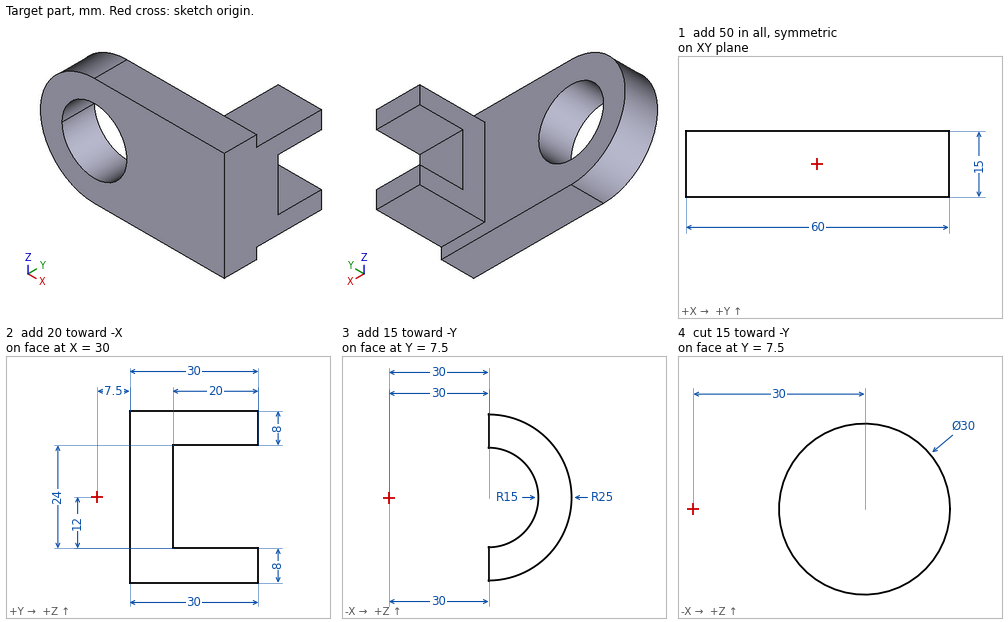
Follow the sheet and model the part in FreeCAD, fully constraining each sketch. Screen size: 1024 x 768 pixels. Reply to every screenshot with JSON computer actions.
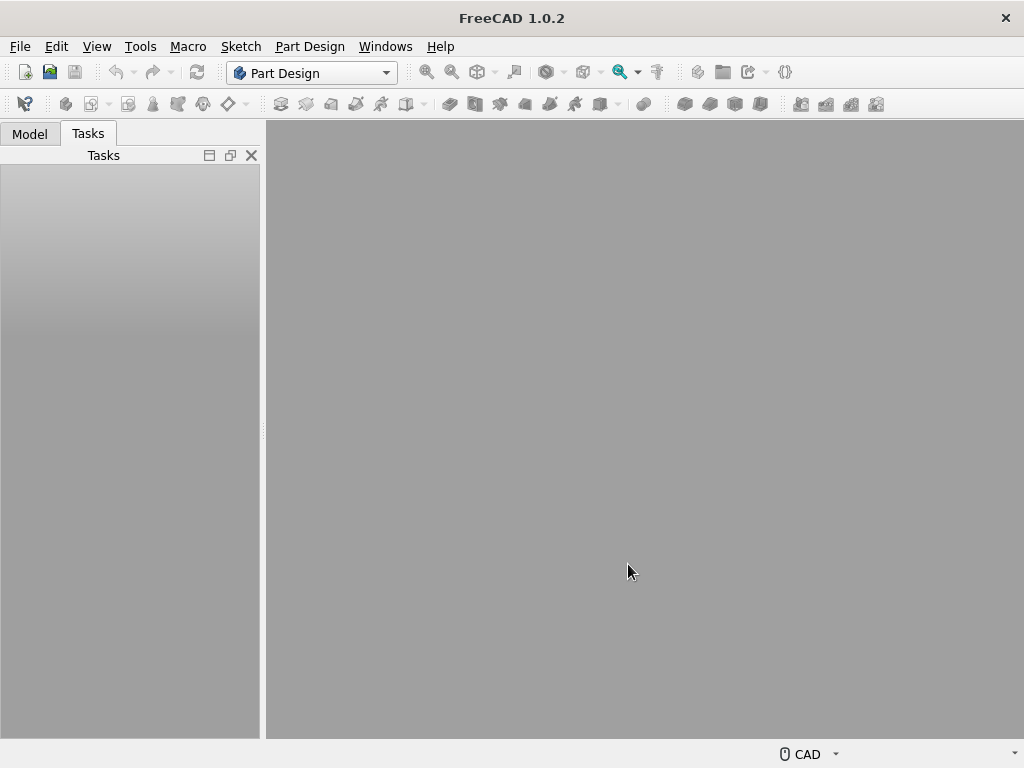
{"action": "left_click", "coordinate": [25, 72]}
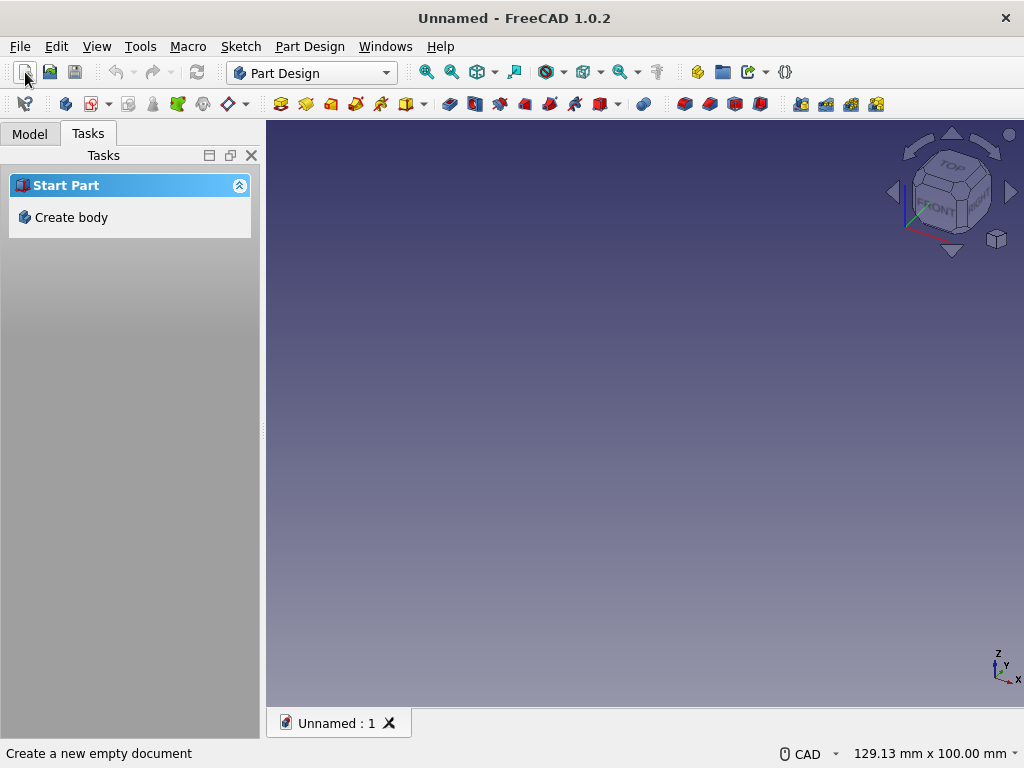
{"action": "left_click", "coordinate": [90, 104]}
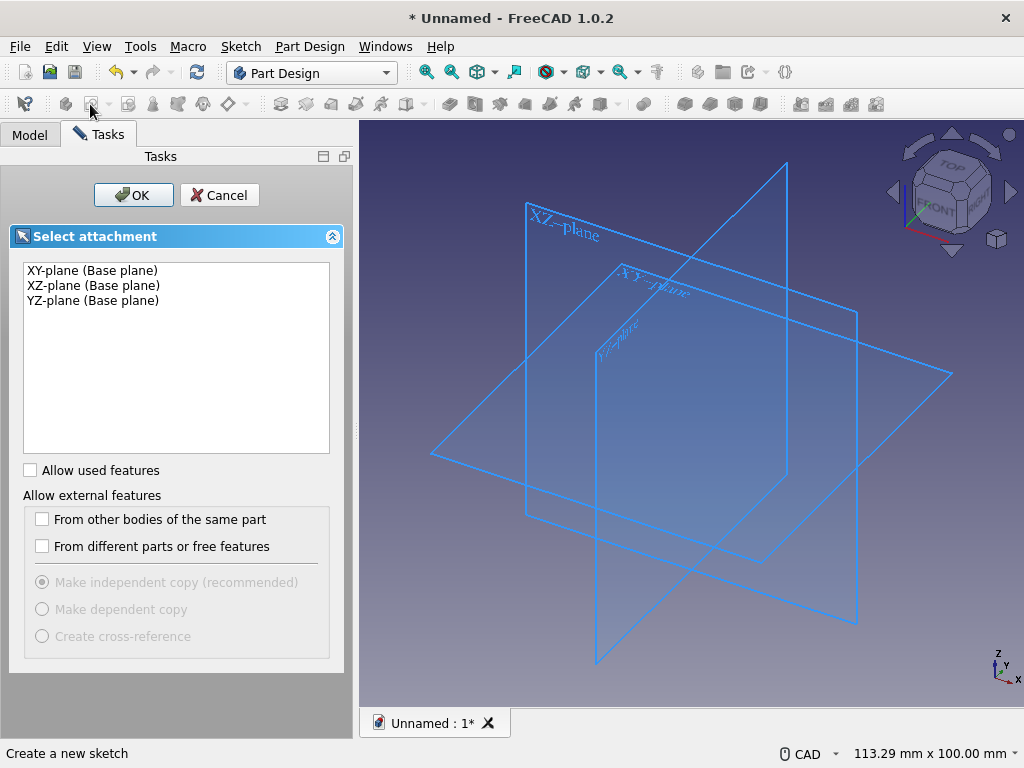
{"action": "left_click", "coordinate": [84, 270]}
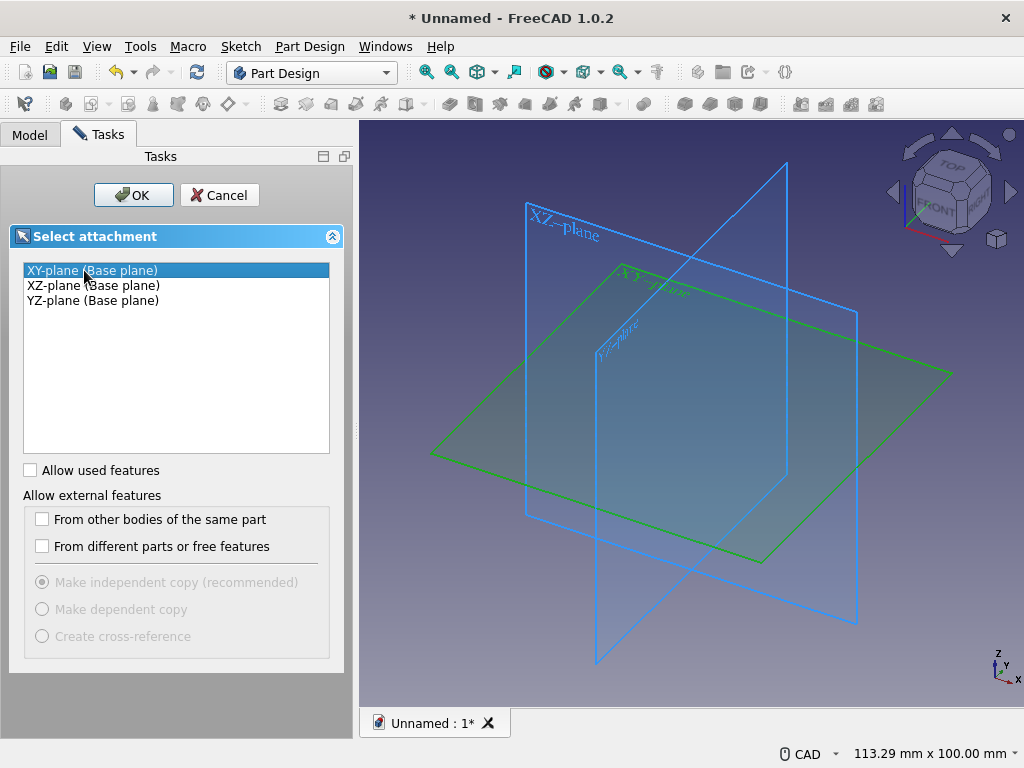
{"action": "left_click", "coordinate": [134, 195]}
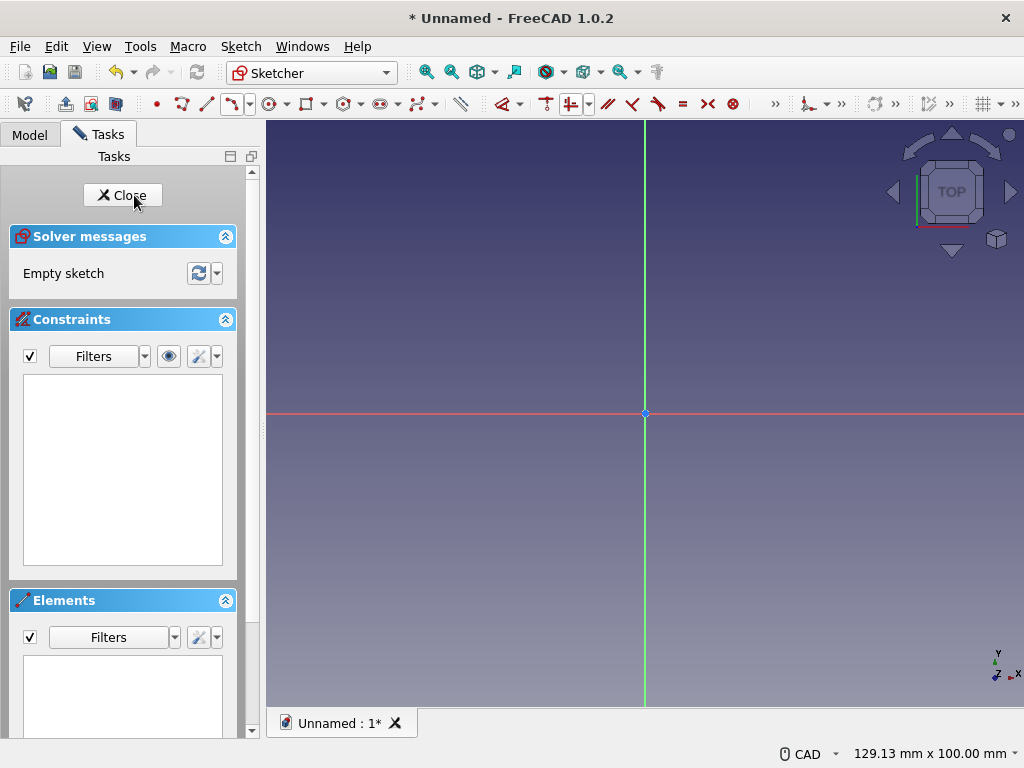
{"action": "key", "text": "g v"}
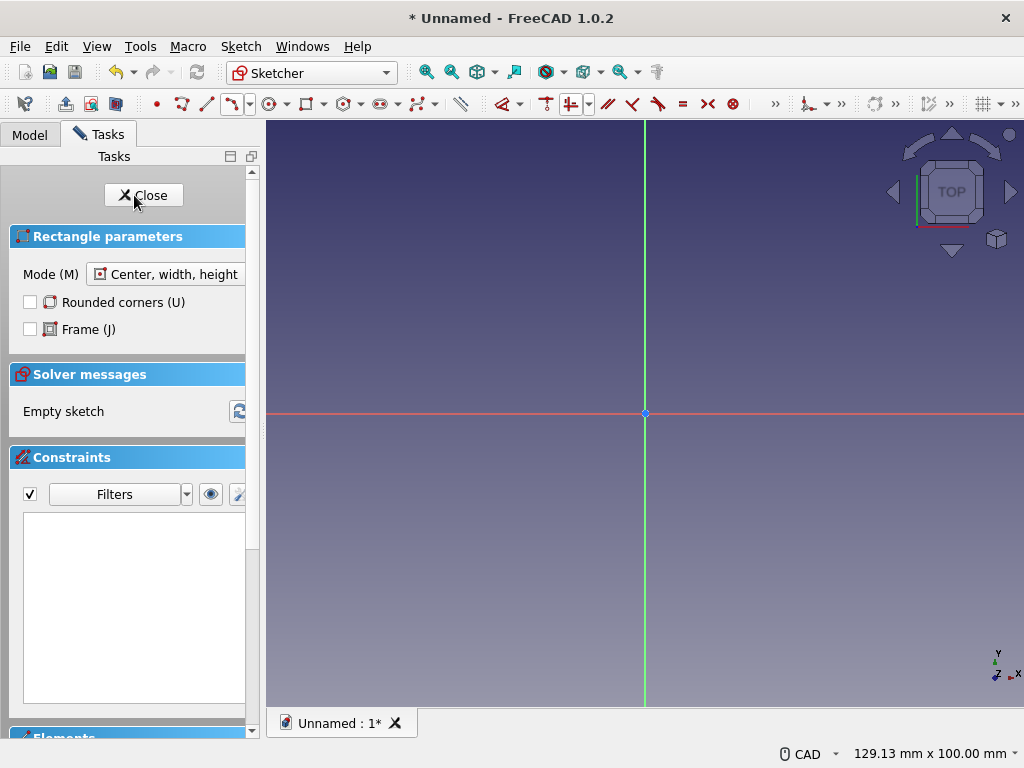
{"action": "left_click", "coordinate": [645, 414]}
{"action": "mouse_move", "coordinate": [821, 369]}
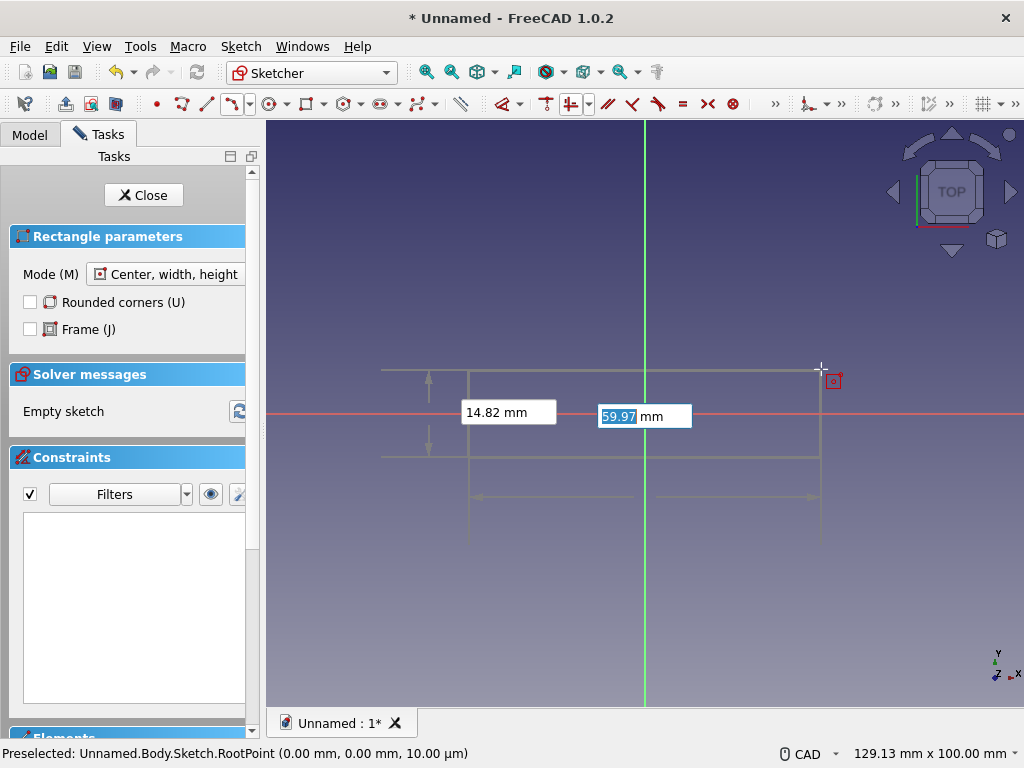
{"action": "type", "text": "60"}
{"action": "key", "text": "Tab"}
{"action": "type", "text": "15"}
{"action": "key", "text": "Return"}
{"action": "key", "text": "Escape"}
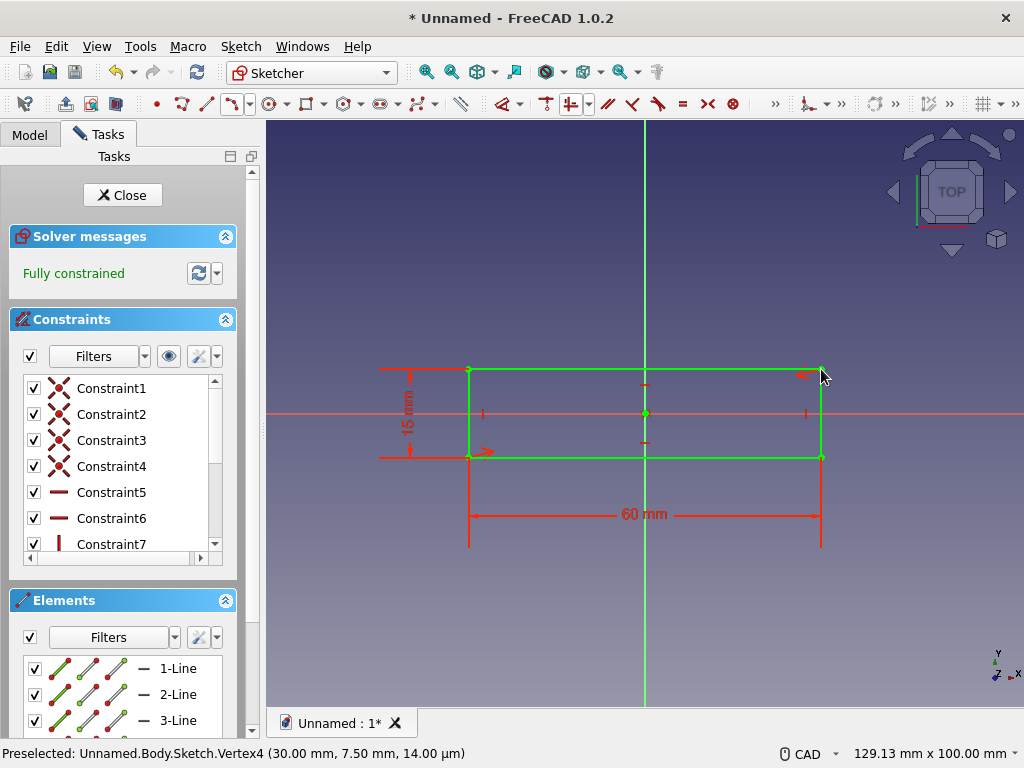
{"action": "left_click", "coordinate": [123, 195]}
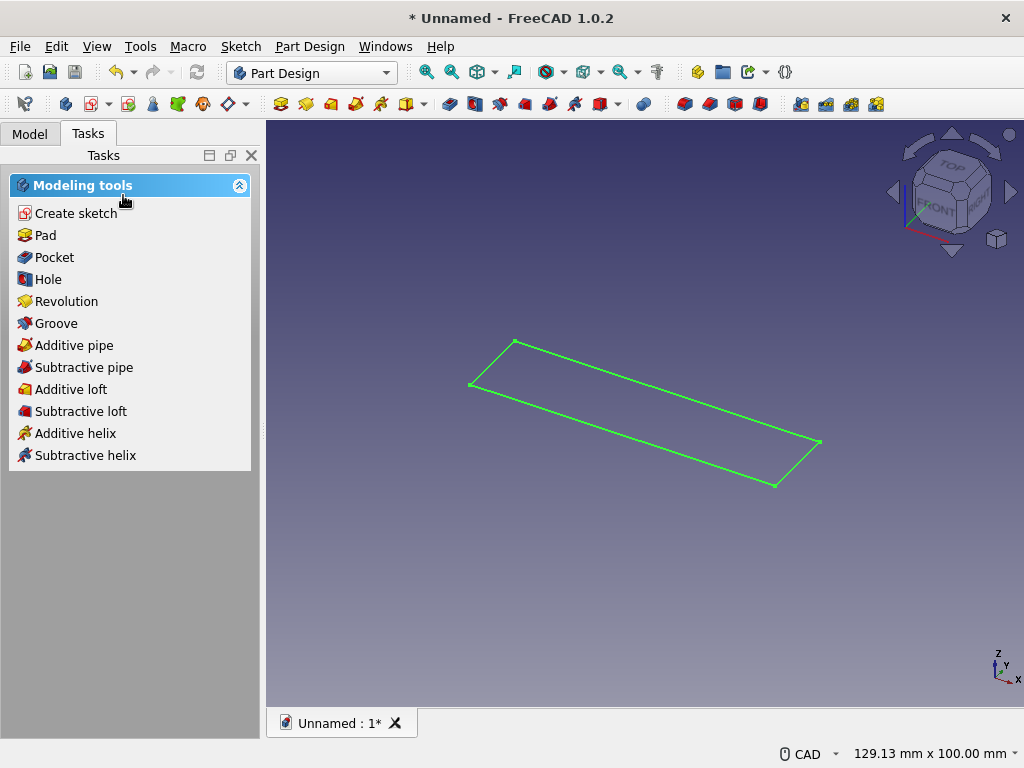
{"action": "left_click", "coordinate": [281, 104]}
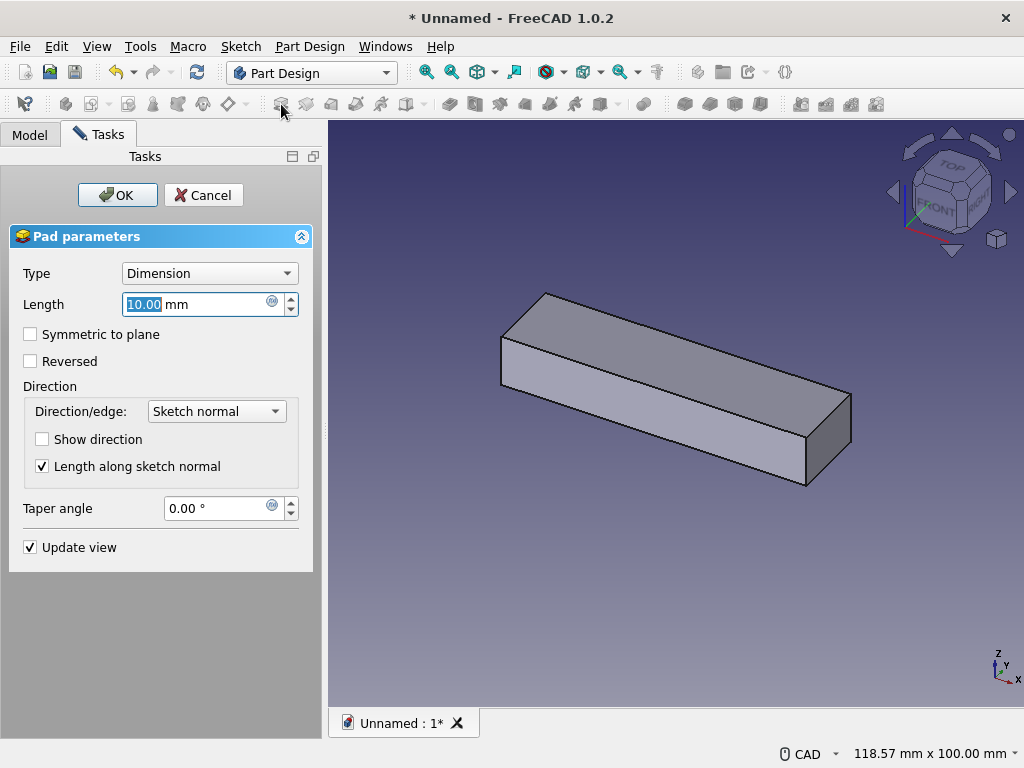
{"action": "type", "text": "50"}
{"action": "key", "text": "Tab"}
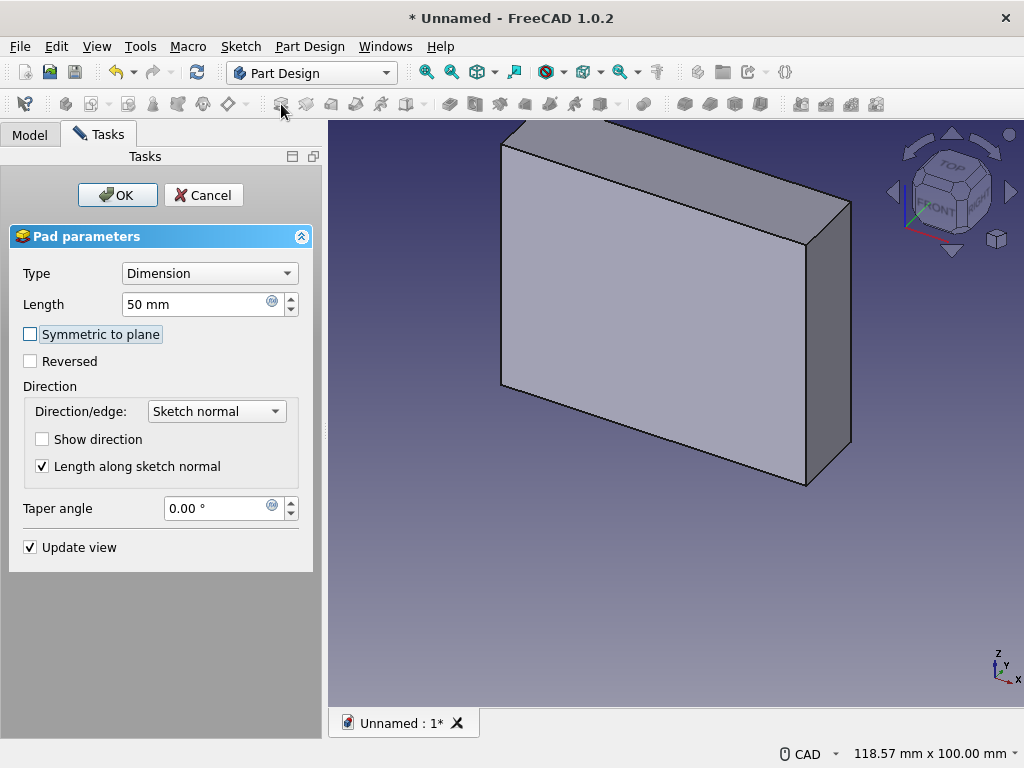
{"action": "left_click", "coordinate": [31, 334]}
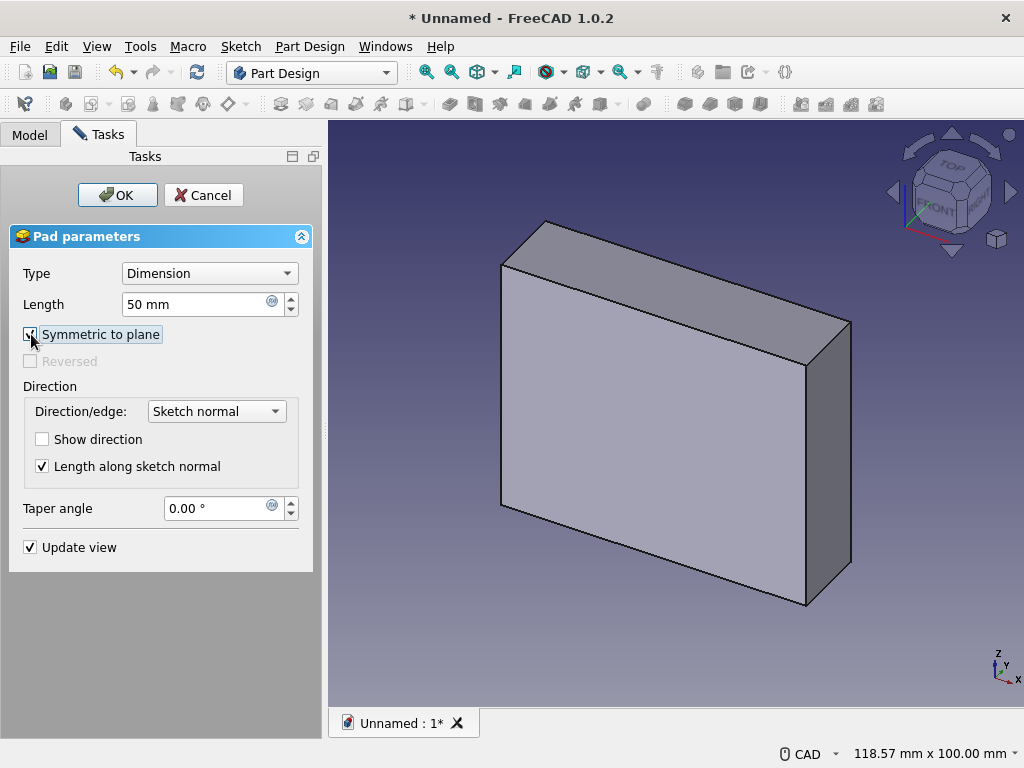
{"action": "left_click", "coordinate": [118, 195]}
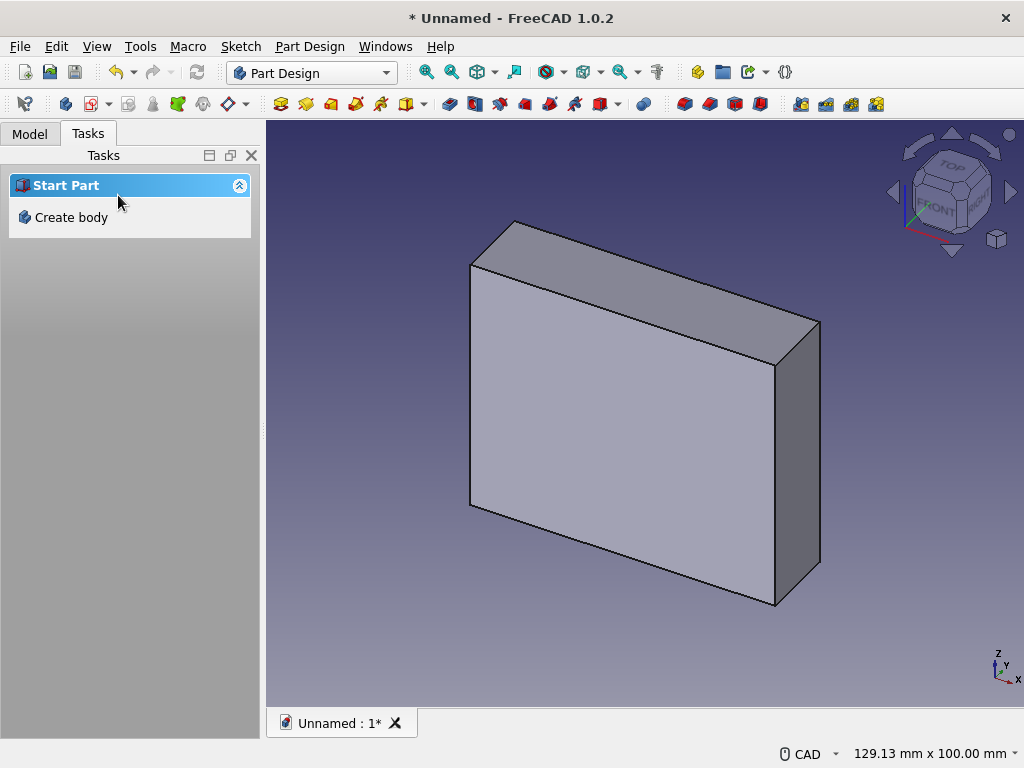
{"action": "left_click", "coordinate": [798, 394]}